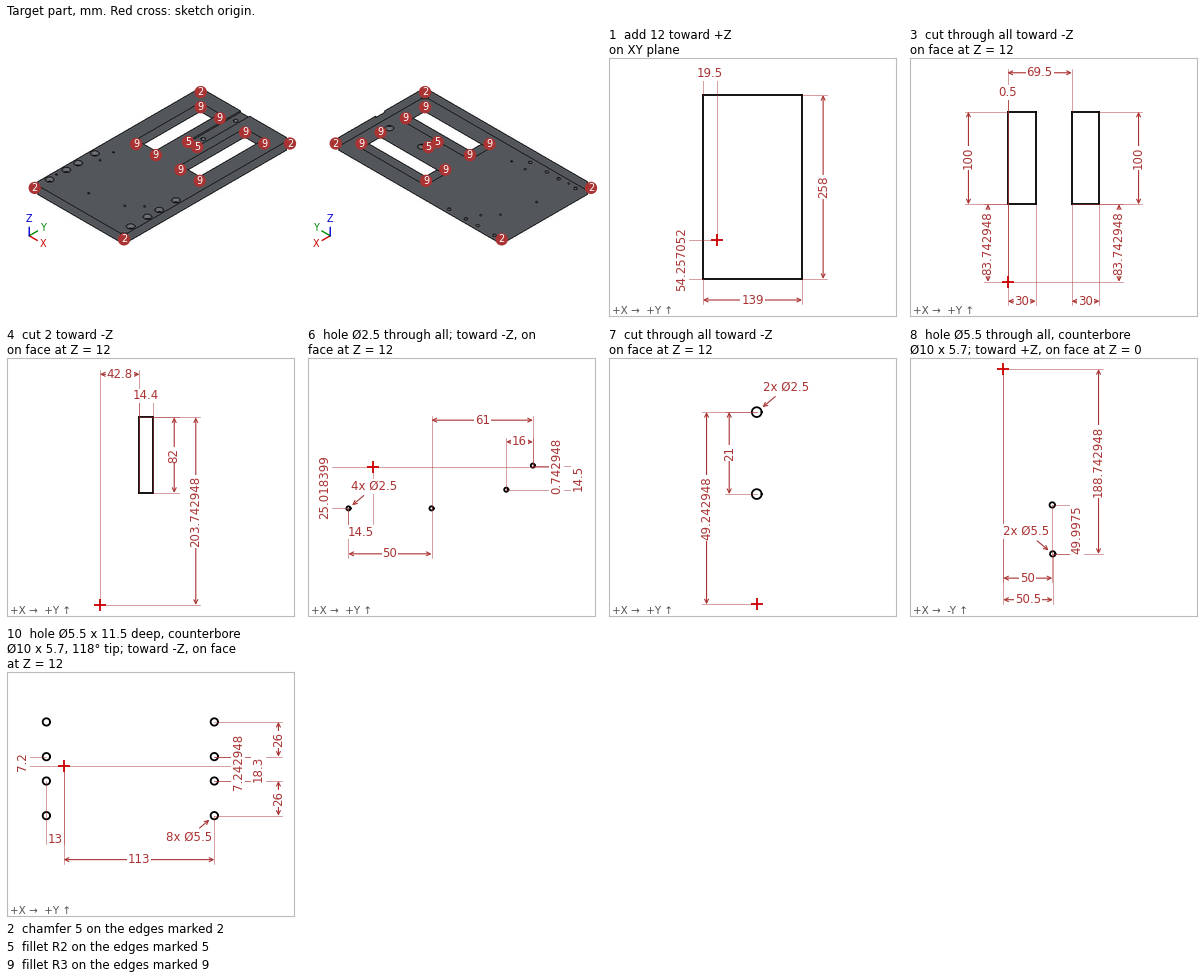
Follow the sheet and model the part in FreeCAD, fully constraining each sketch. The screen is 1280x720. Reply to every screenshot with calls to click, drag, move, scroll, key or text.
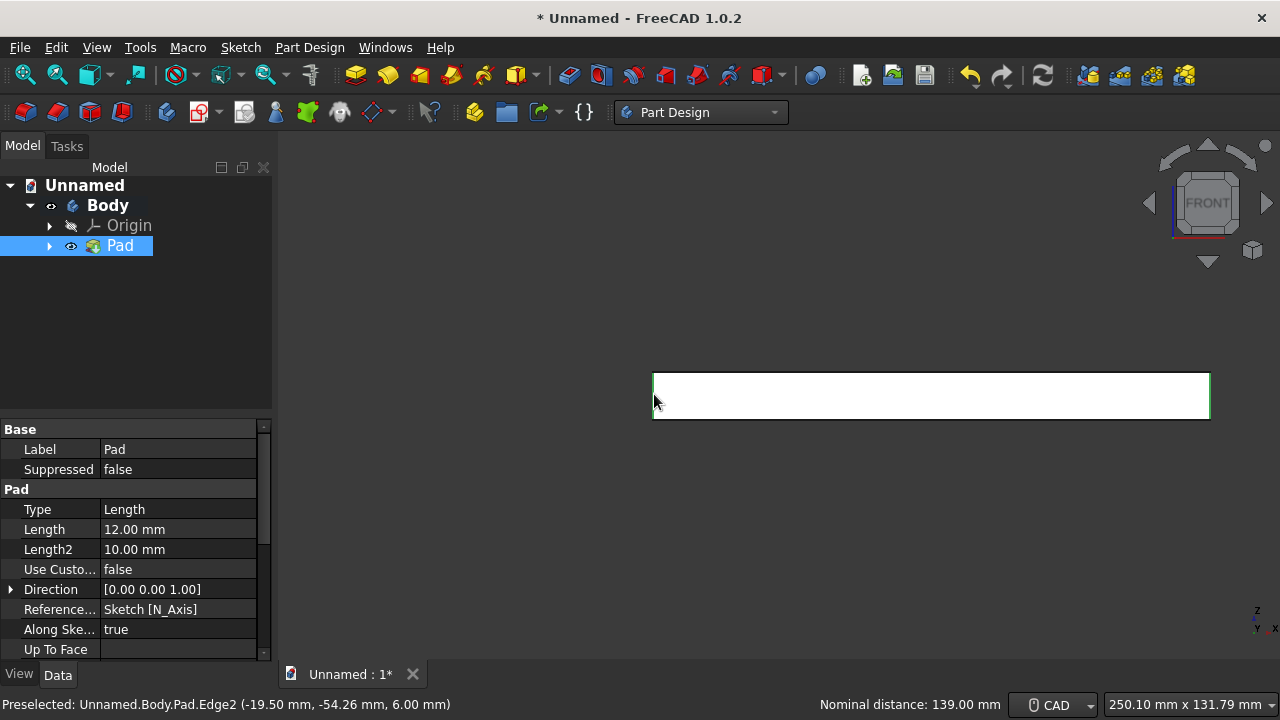
click(26, 76)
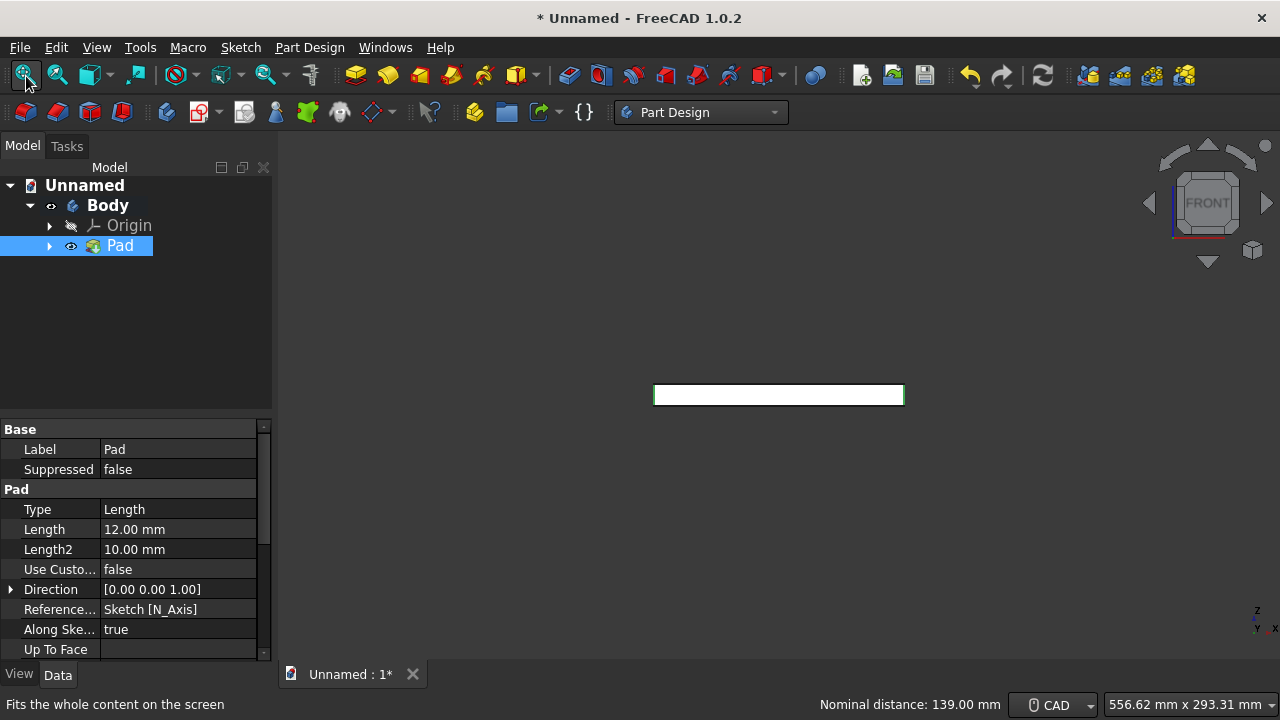
key(3)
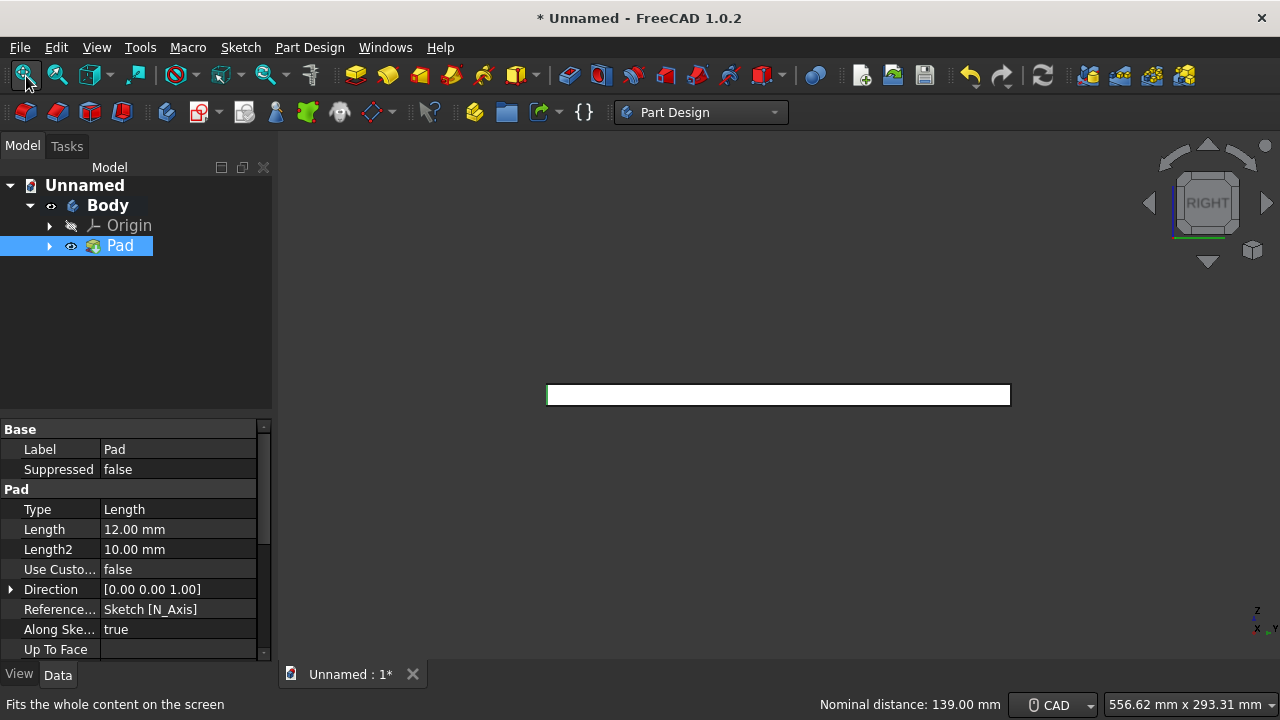
click(1011, 394, ctrl)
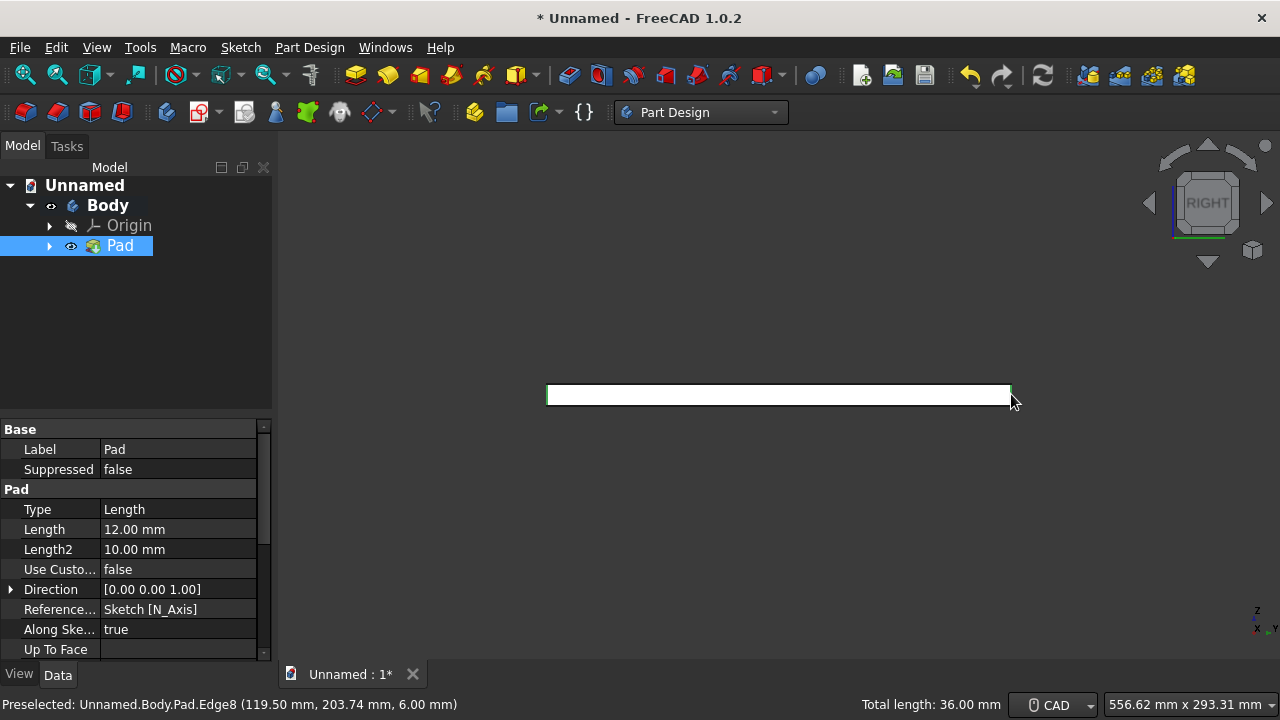
scroll(1011, 394, up, 4)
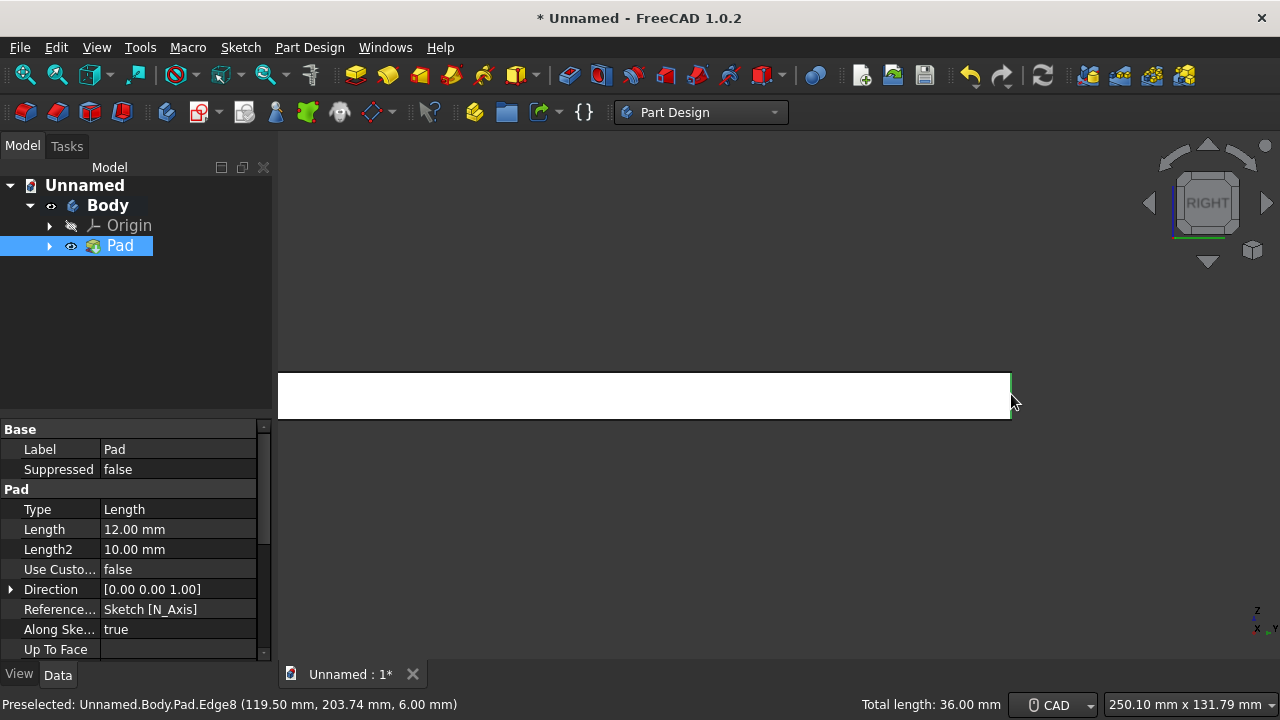
key(v)
key(f)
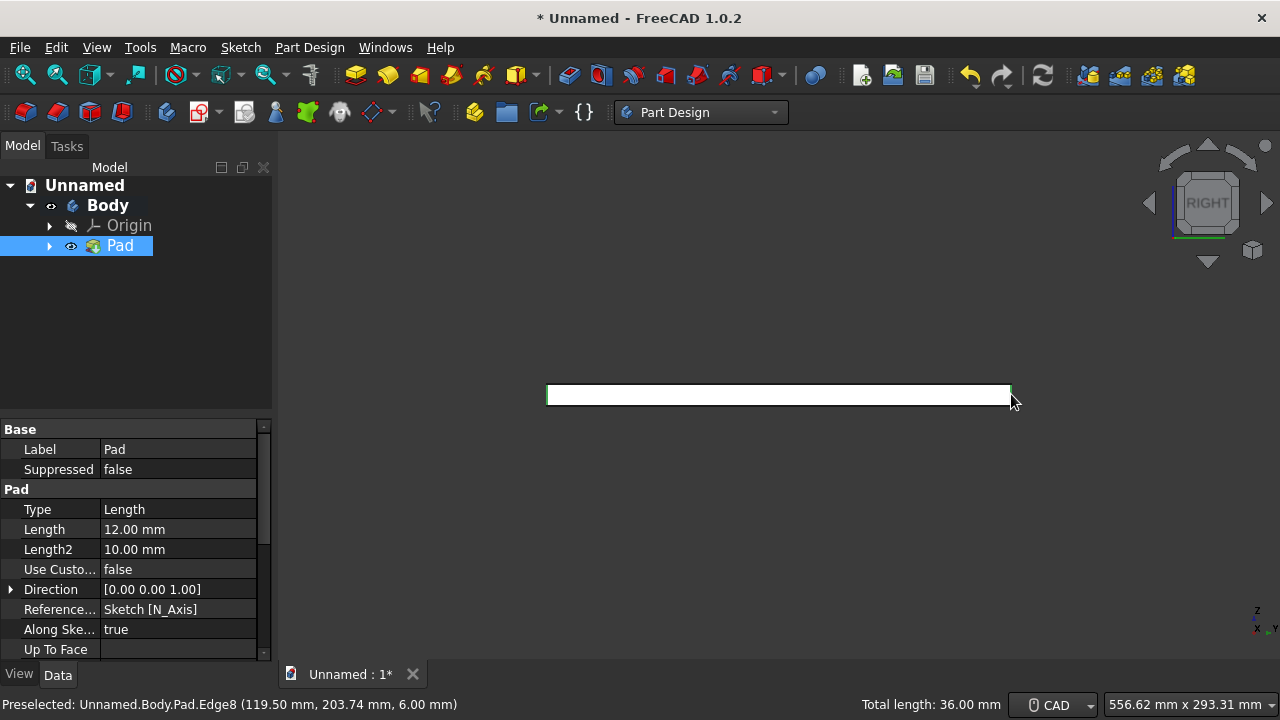
key(5)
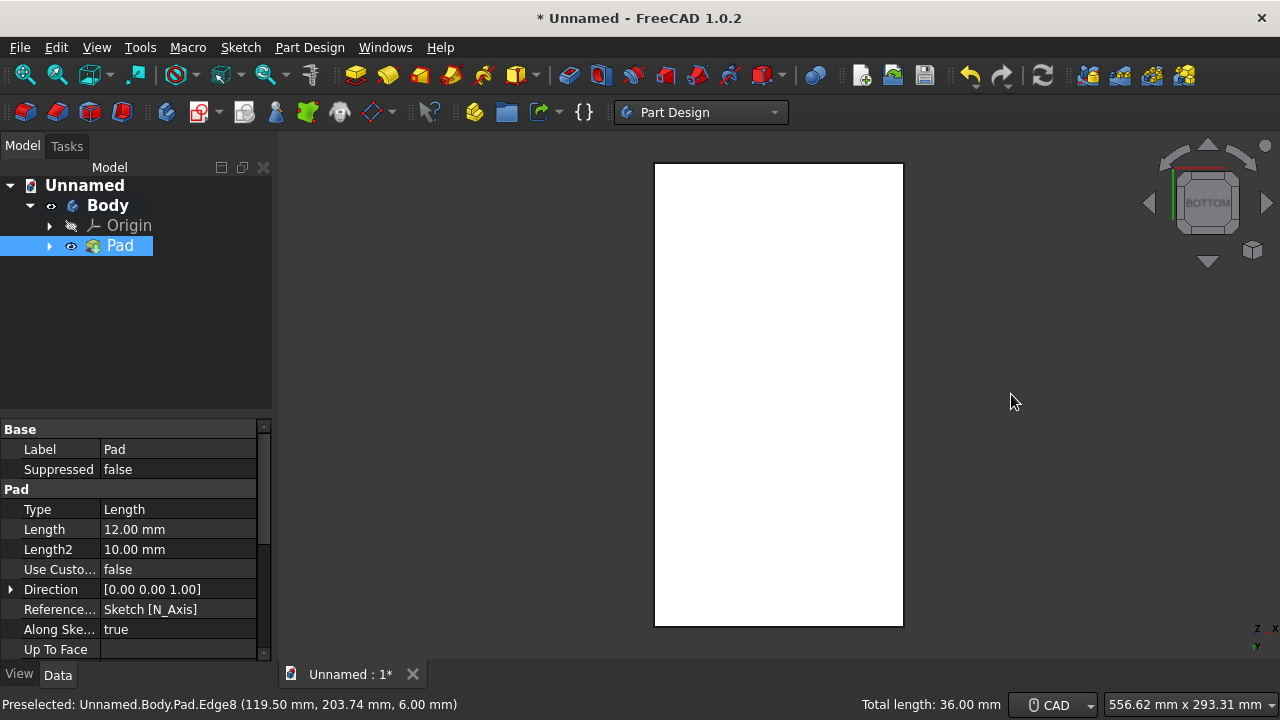
scroll(654, 626, up, 4)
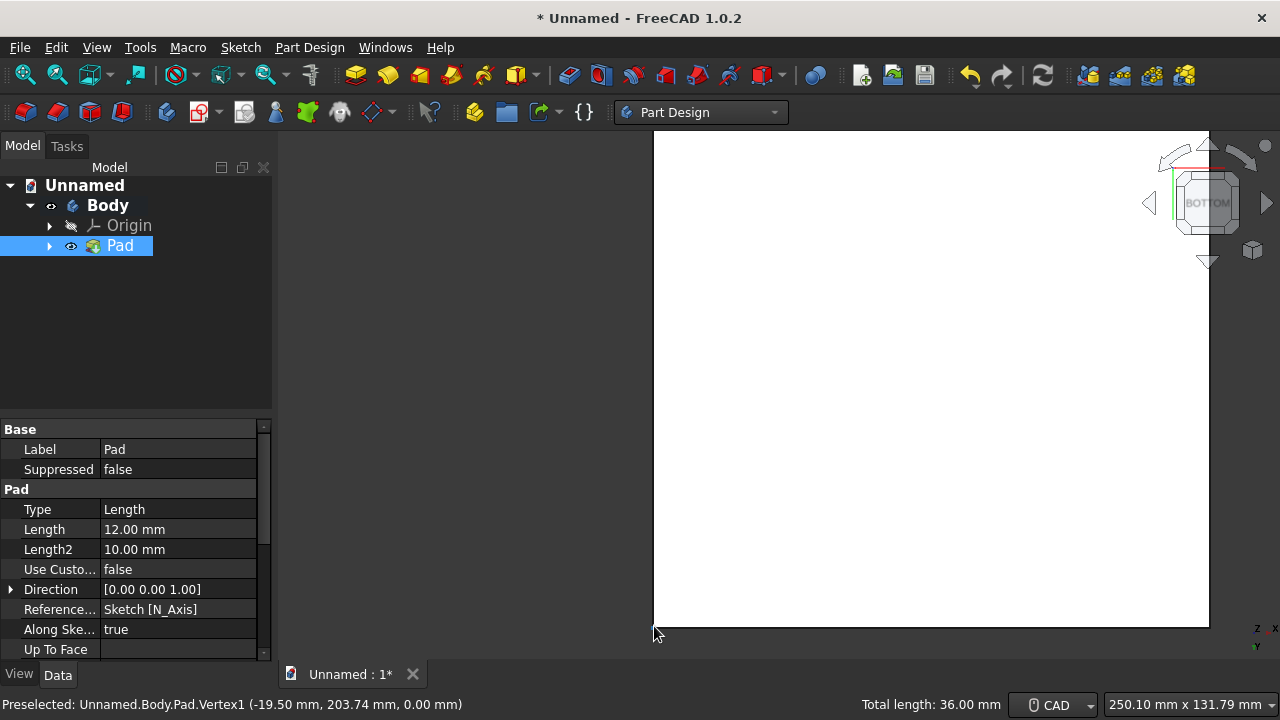
click(26, 76)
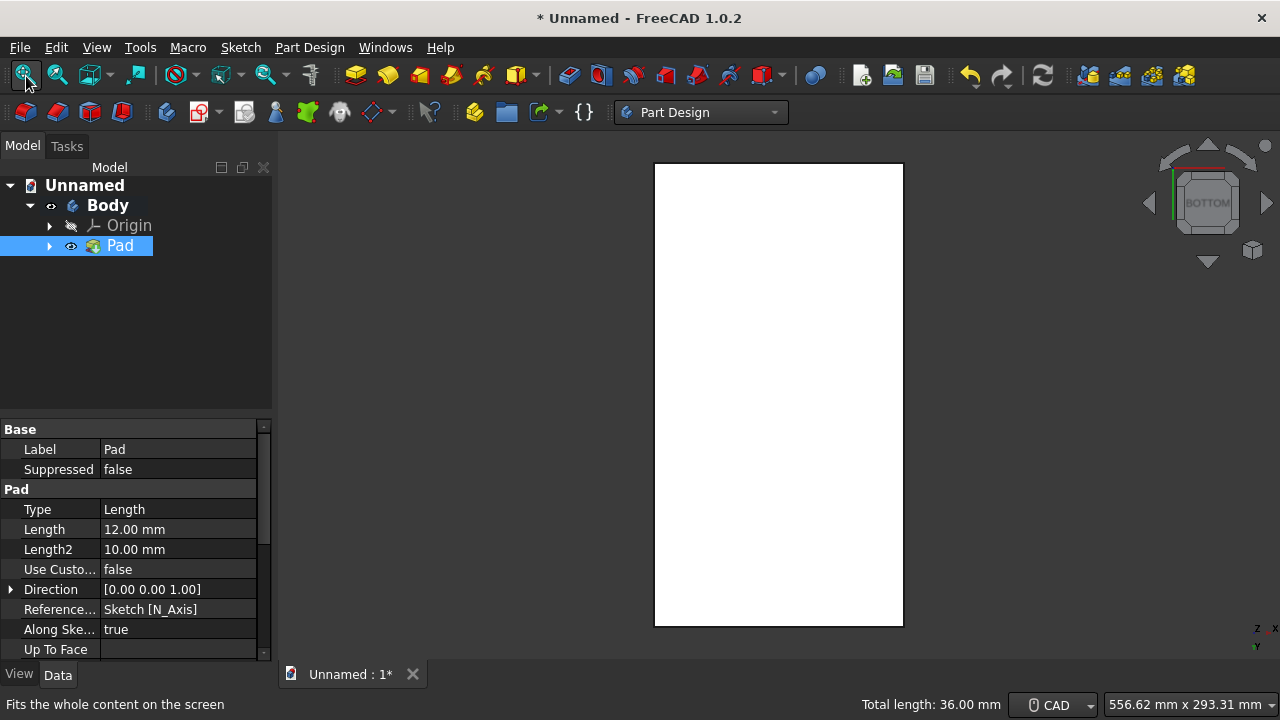
key(4)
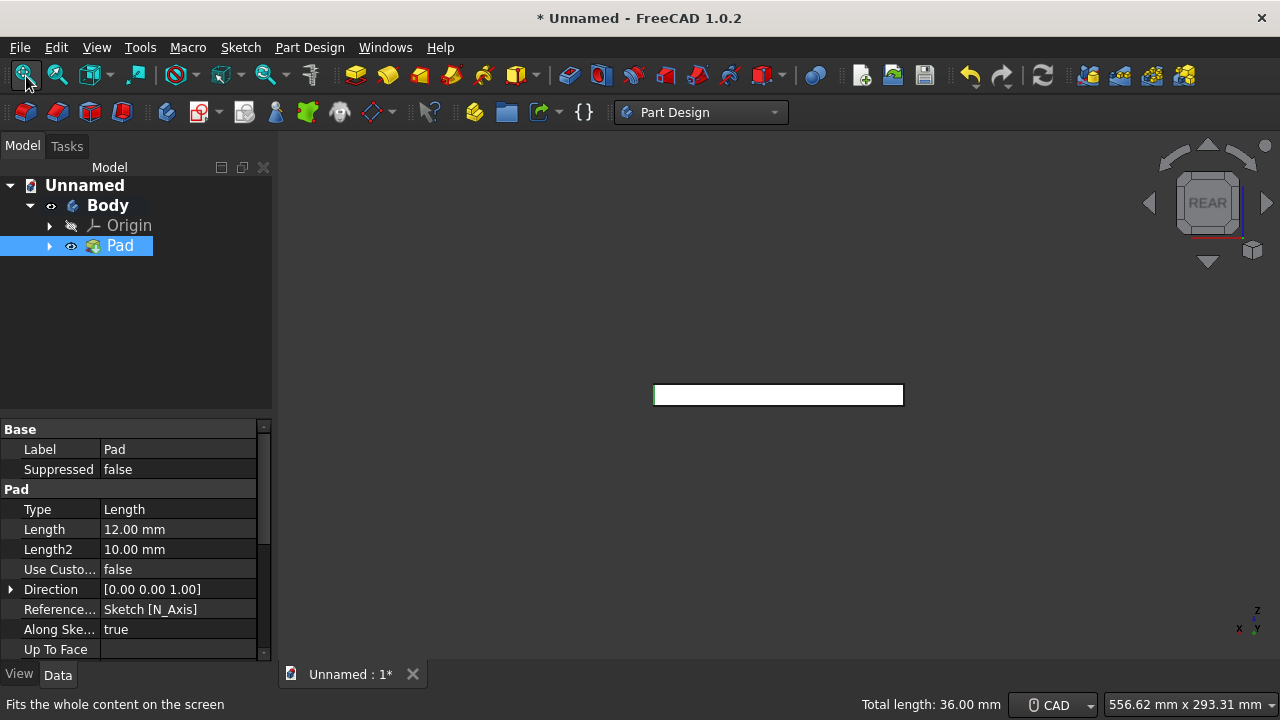
key(v)
key(f)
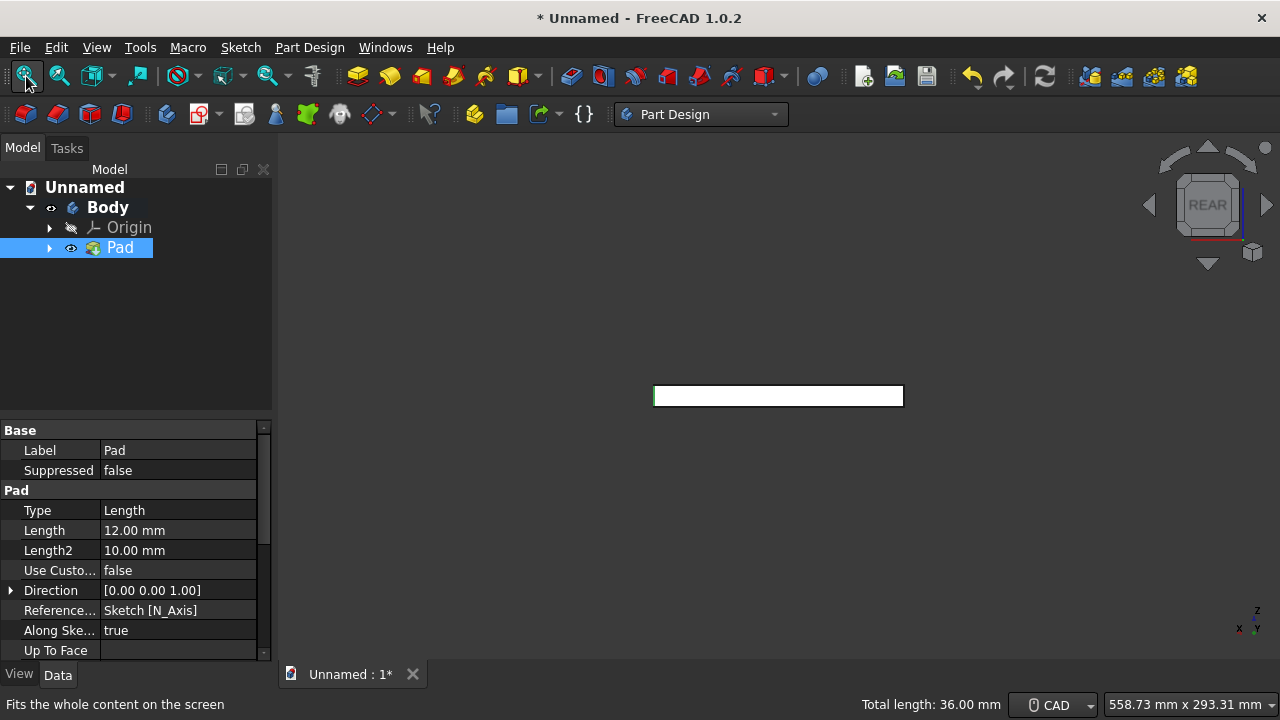
click(904, 395, ctrl)